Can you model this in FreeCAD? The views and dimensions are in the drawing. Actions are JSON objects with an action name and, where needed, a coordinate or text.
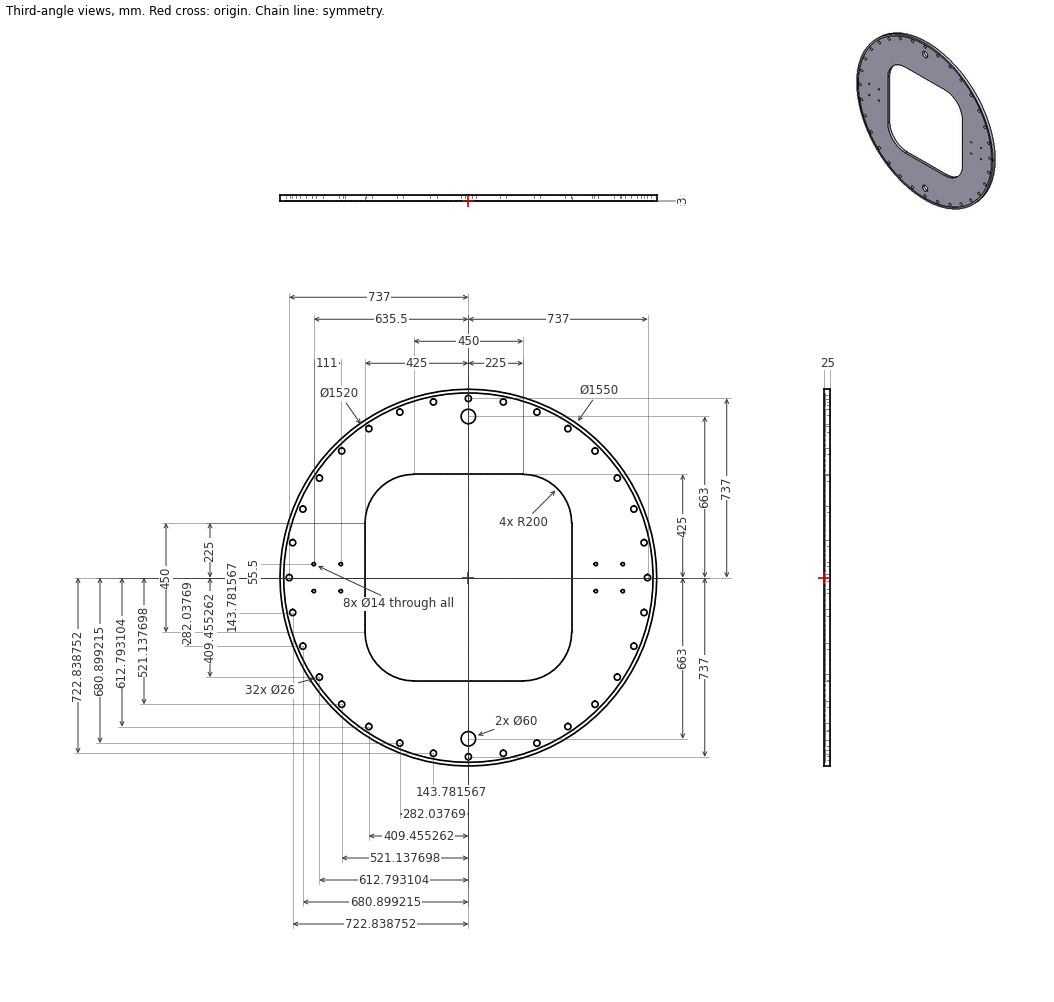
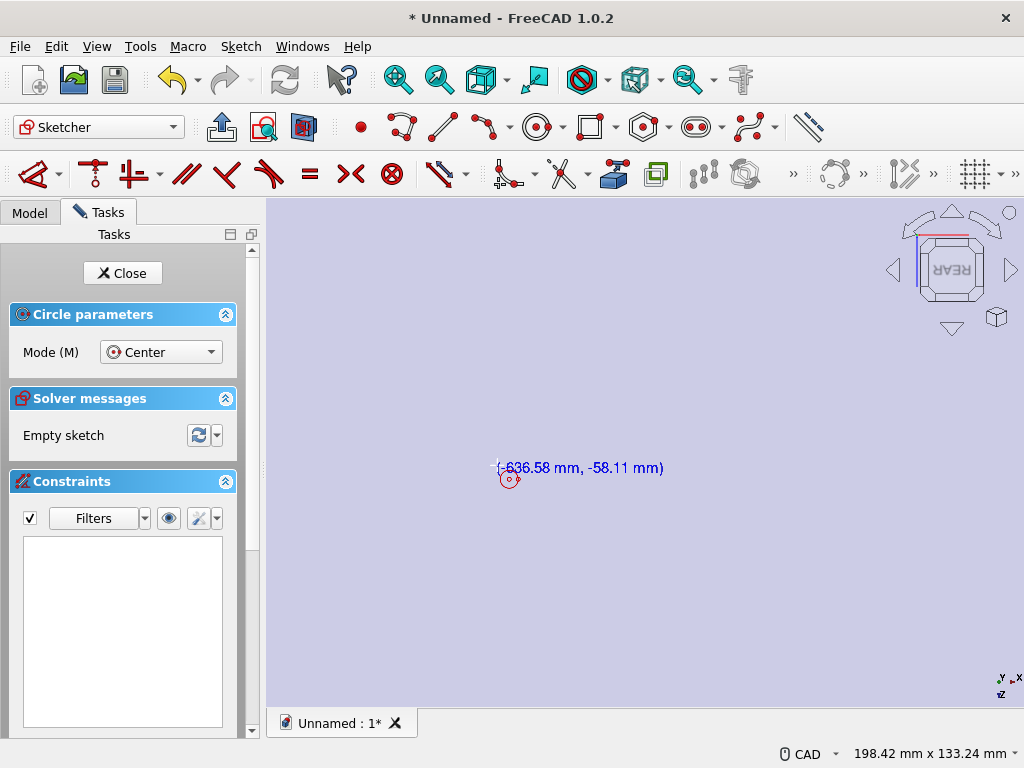
{"action": "scroll", "coordinate": [388, 469], "scroll_direction": "down", "scroll_amount": 13}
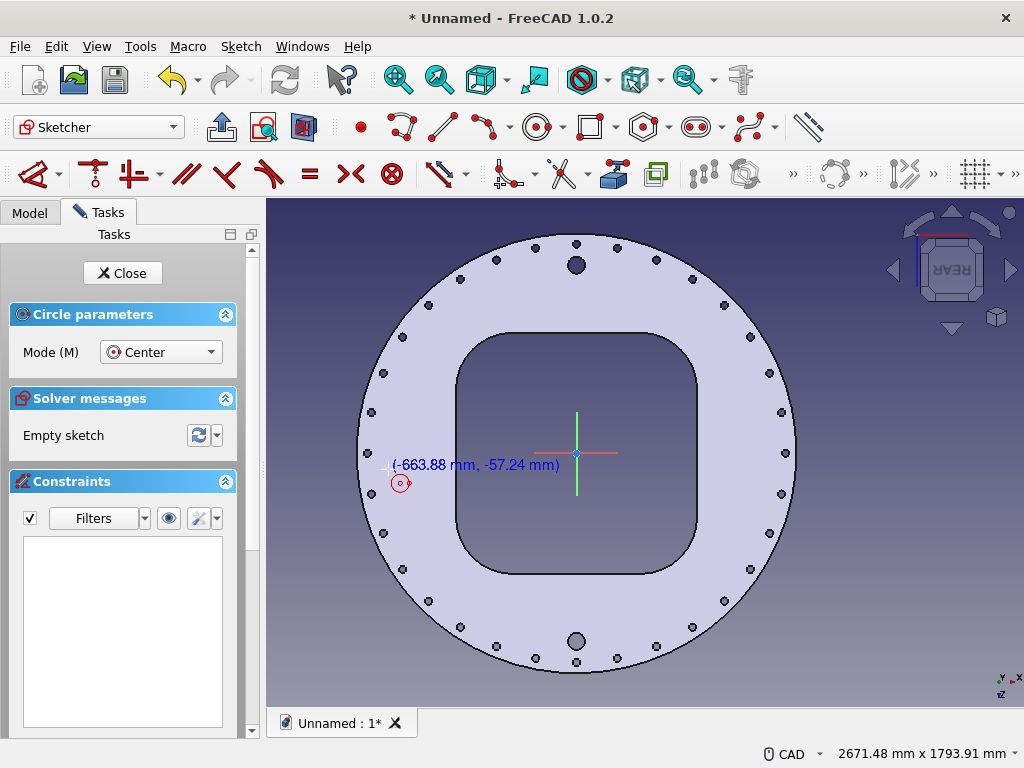
{"action": "left_click", "coordinate": [396, 469]}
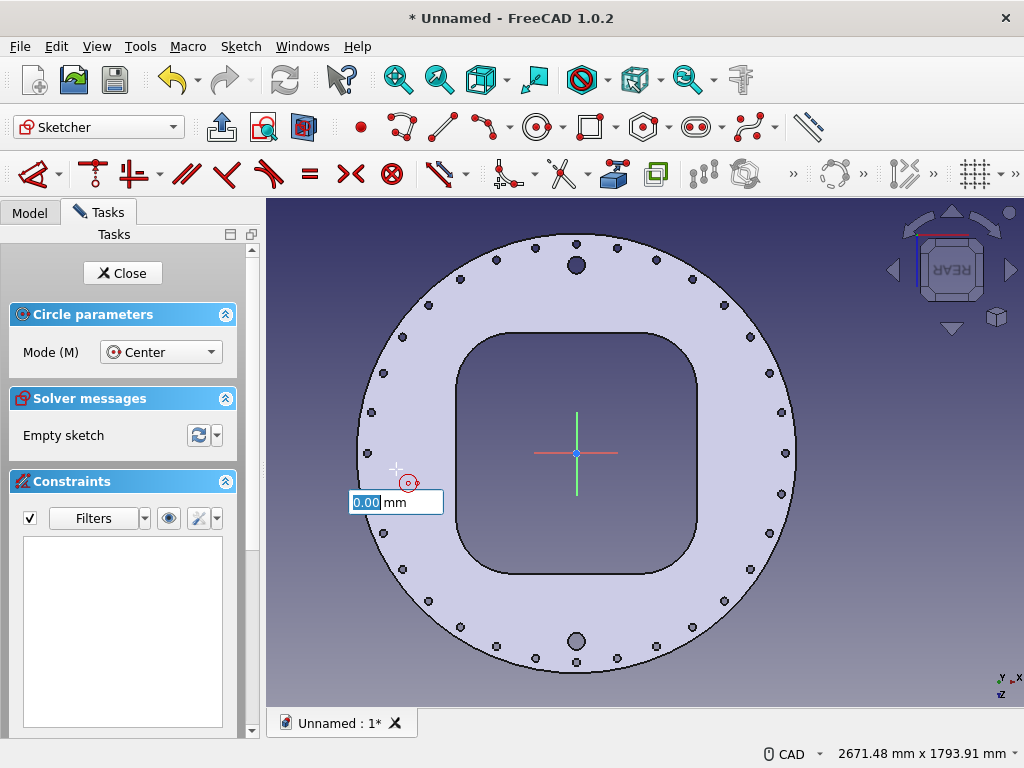
{"action": "scroll", "coordinate": [398, 468], "scroll_direction": "up", "scroll_amount": 11}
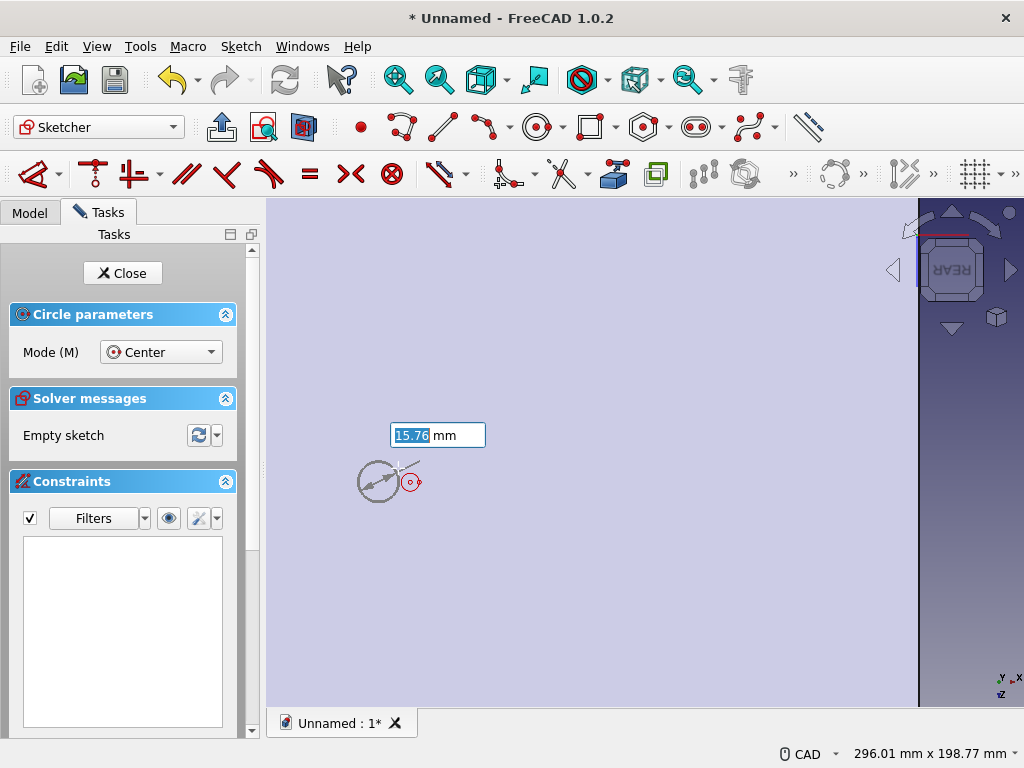
{"action": "left_click", "coordinate": [393, 461]}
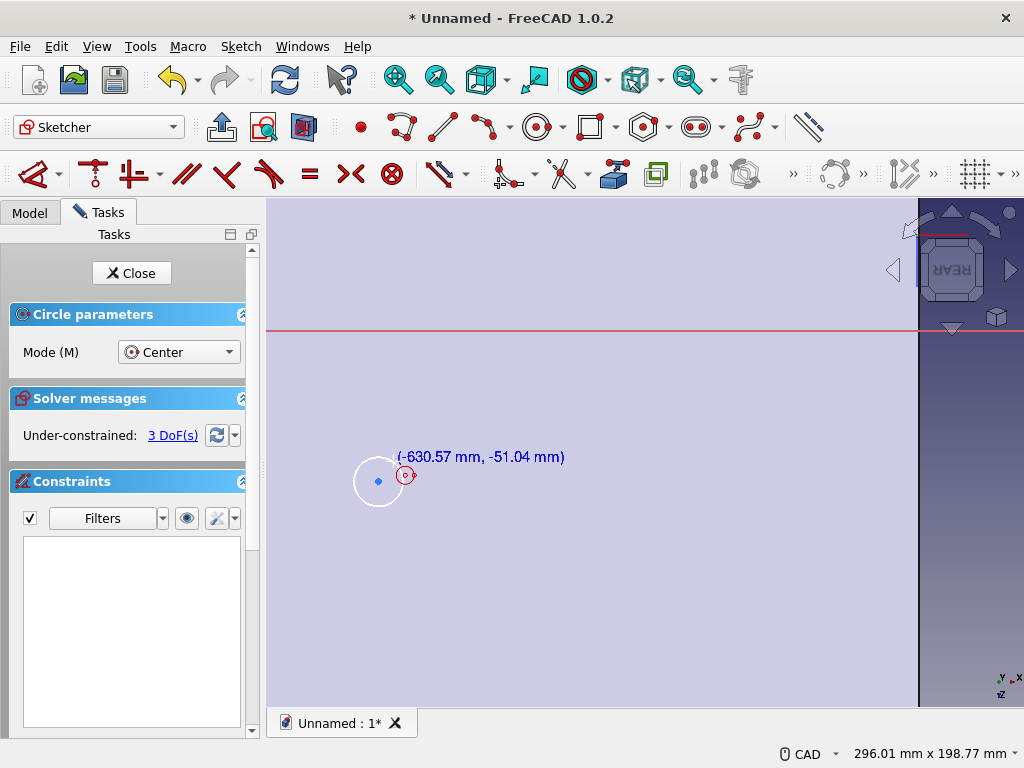
{"action": "scroll", "coordinate": [665, 473], "scroll_direction": "up", "scroll_amount": 2}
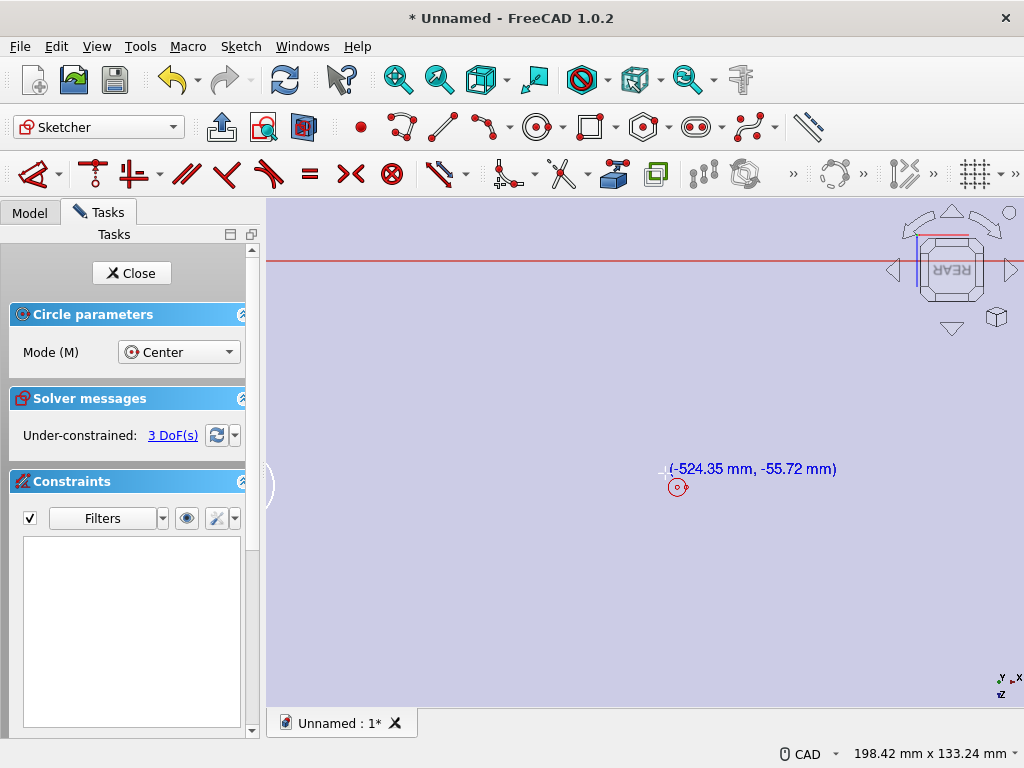
{"action": "scroll", "coordinate": [409, 468], "scroll_direction": "down", "scroll_amount": 13}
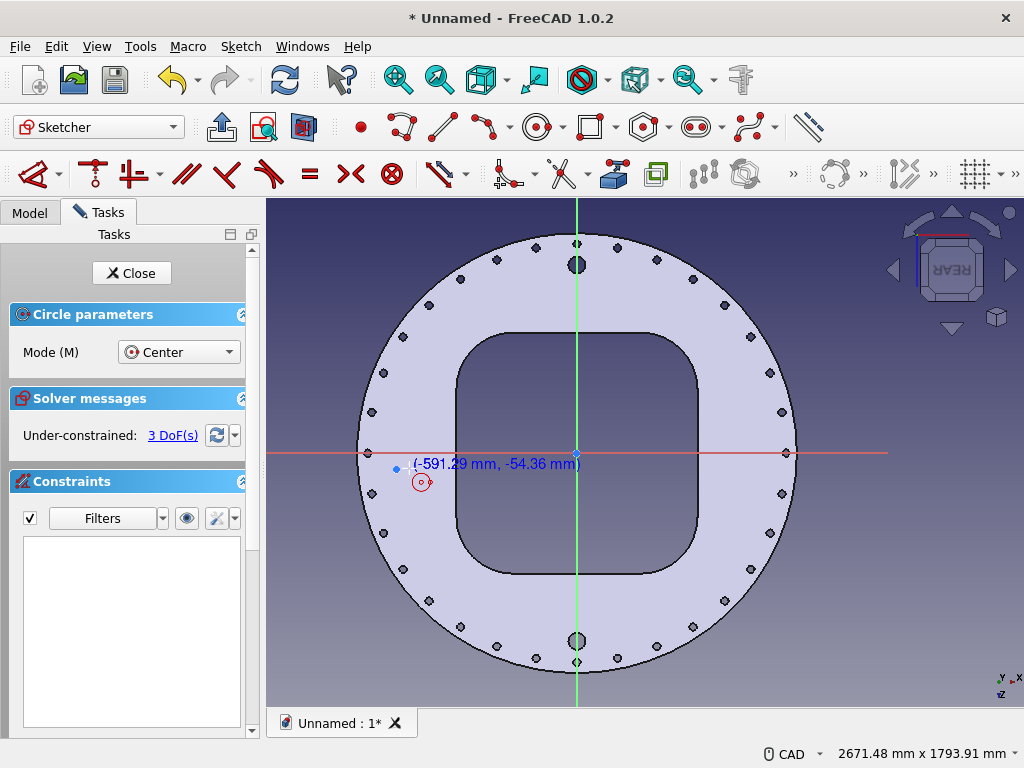
{"action": "left_click", "coordinate": [428, 469]}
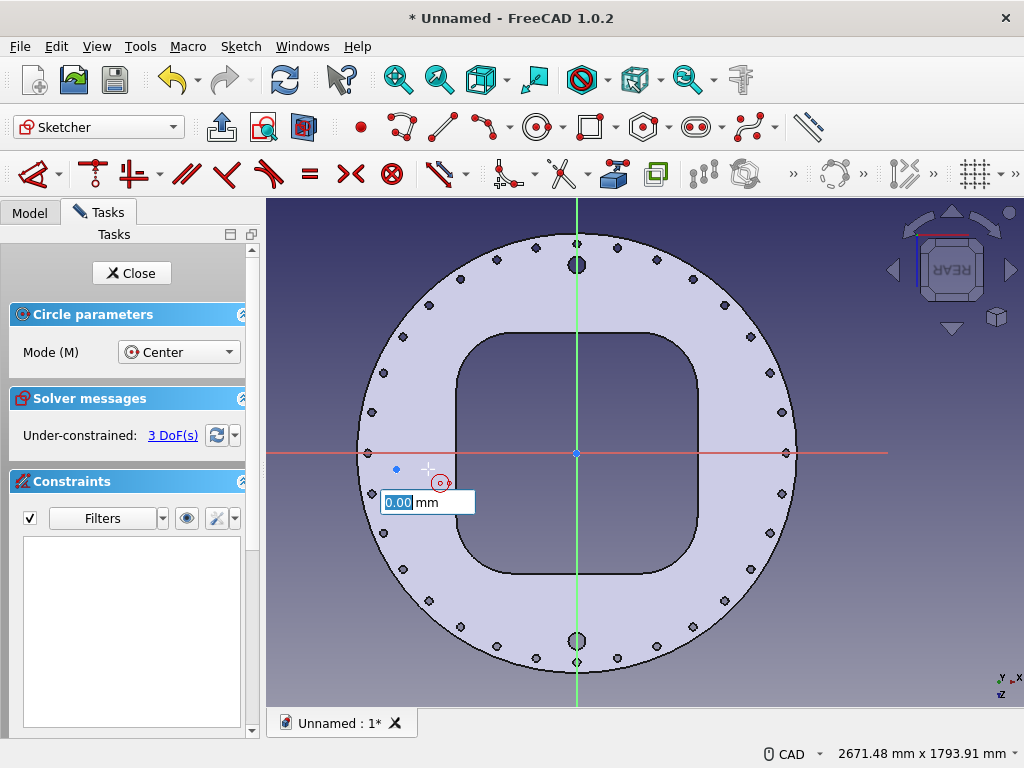
{"action": "scroll", "coordinate": [430, 467], "scroll_direction": "up", "scroll_amount": 11}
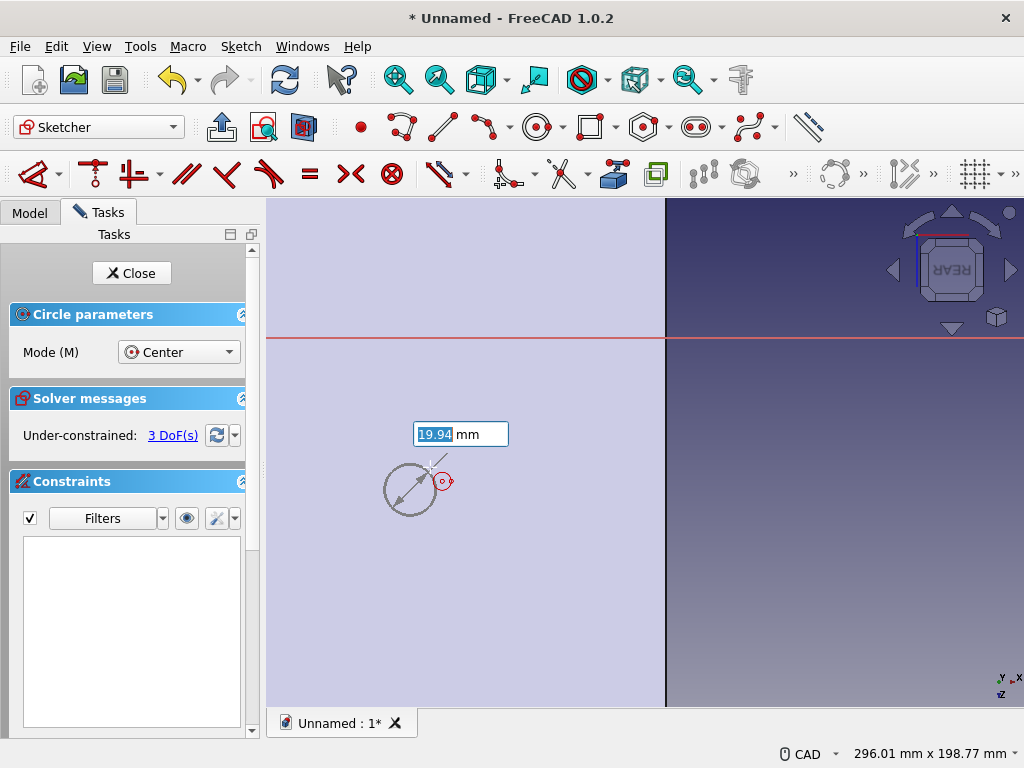
{"action": "left_click", "coordinate": [424, 467]}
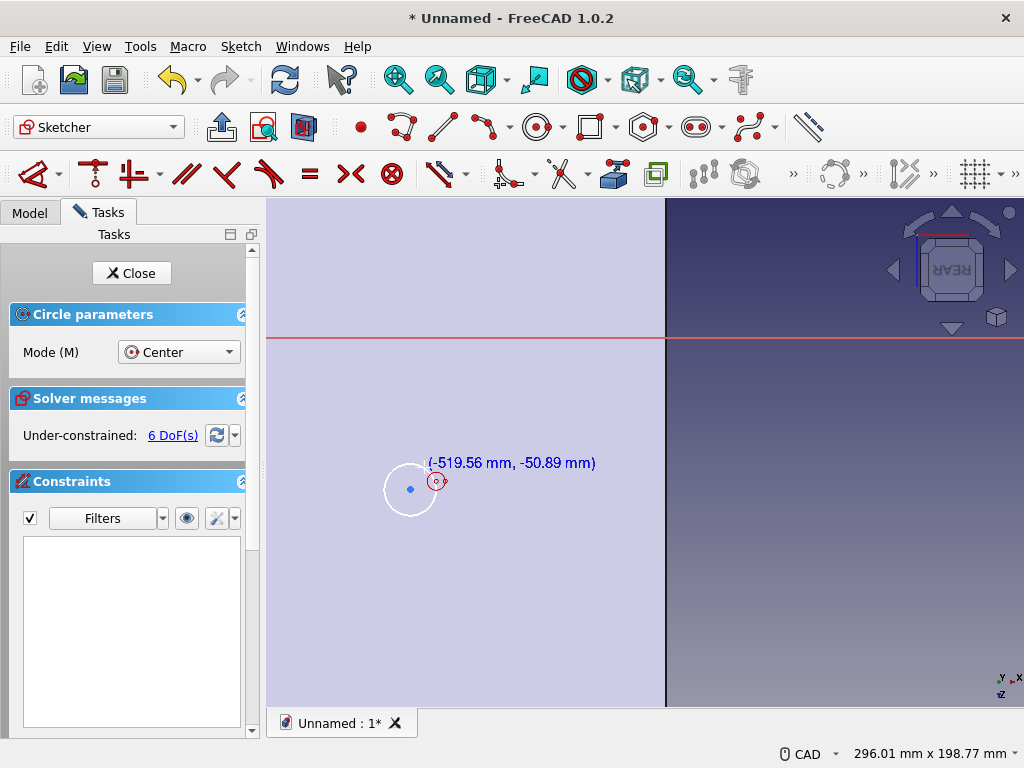
{"action": "scroll", "coordinate": [430, 467], "scroll_direction": "down", "scroll_amount": 11}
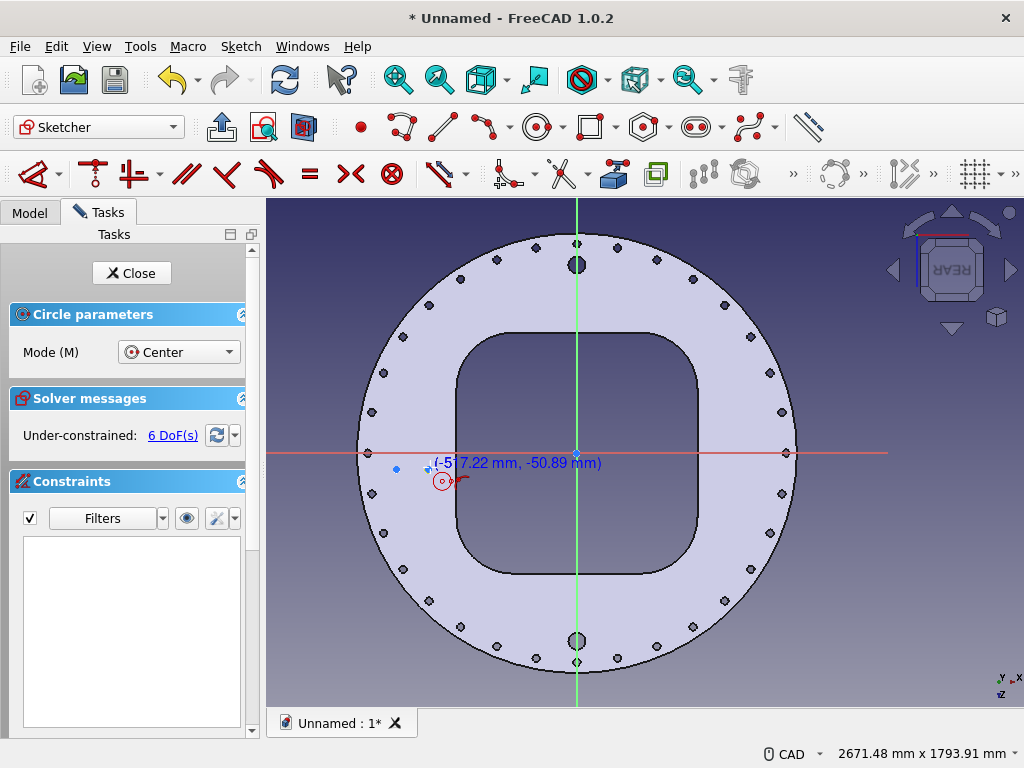
{"action": "scroll", "coordinate": [428, 437], "scroll_direction": "up", "scroll_amount": 13}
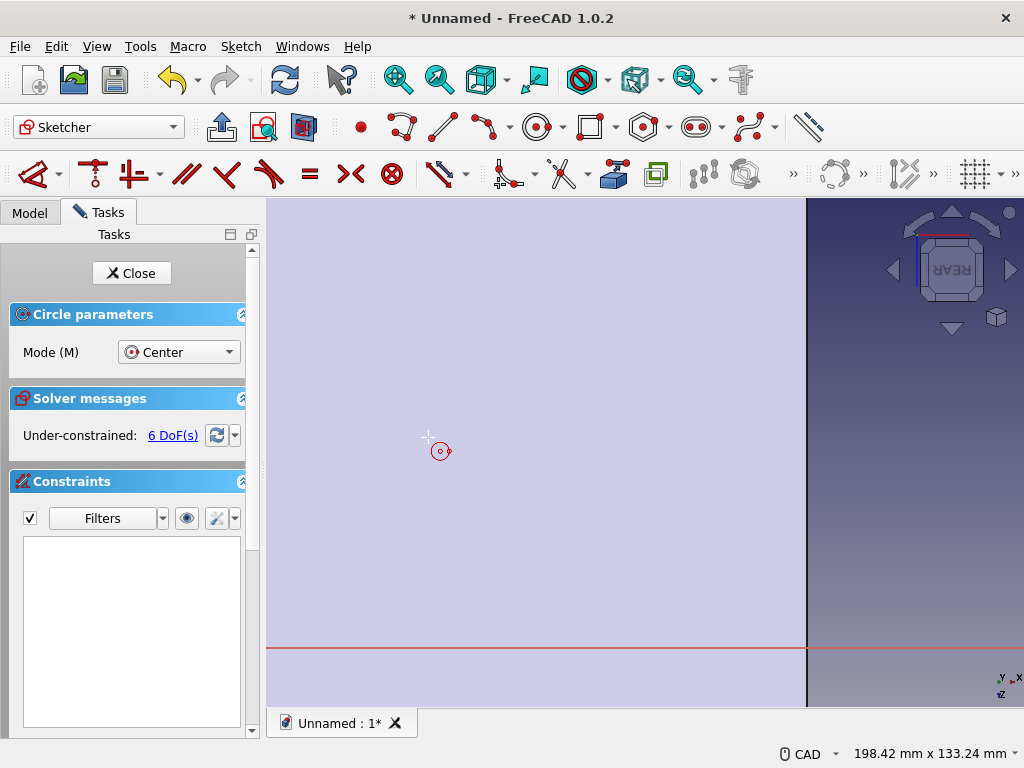
{"action": "scroll", "coordinate": [428, 437], "scroll_direction": "down", "scroll_amount": 13}